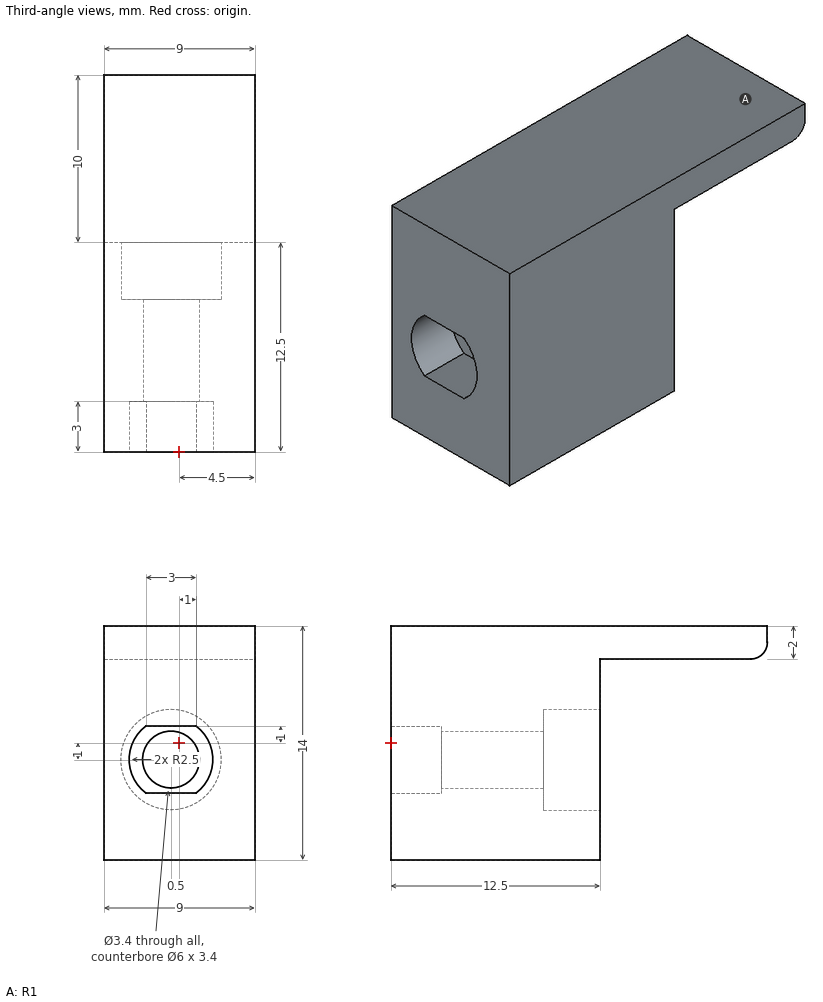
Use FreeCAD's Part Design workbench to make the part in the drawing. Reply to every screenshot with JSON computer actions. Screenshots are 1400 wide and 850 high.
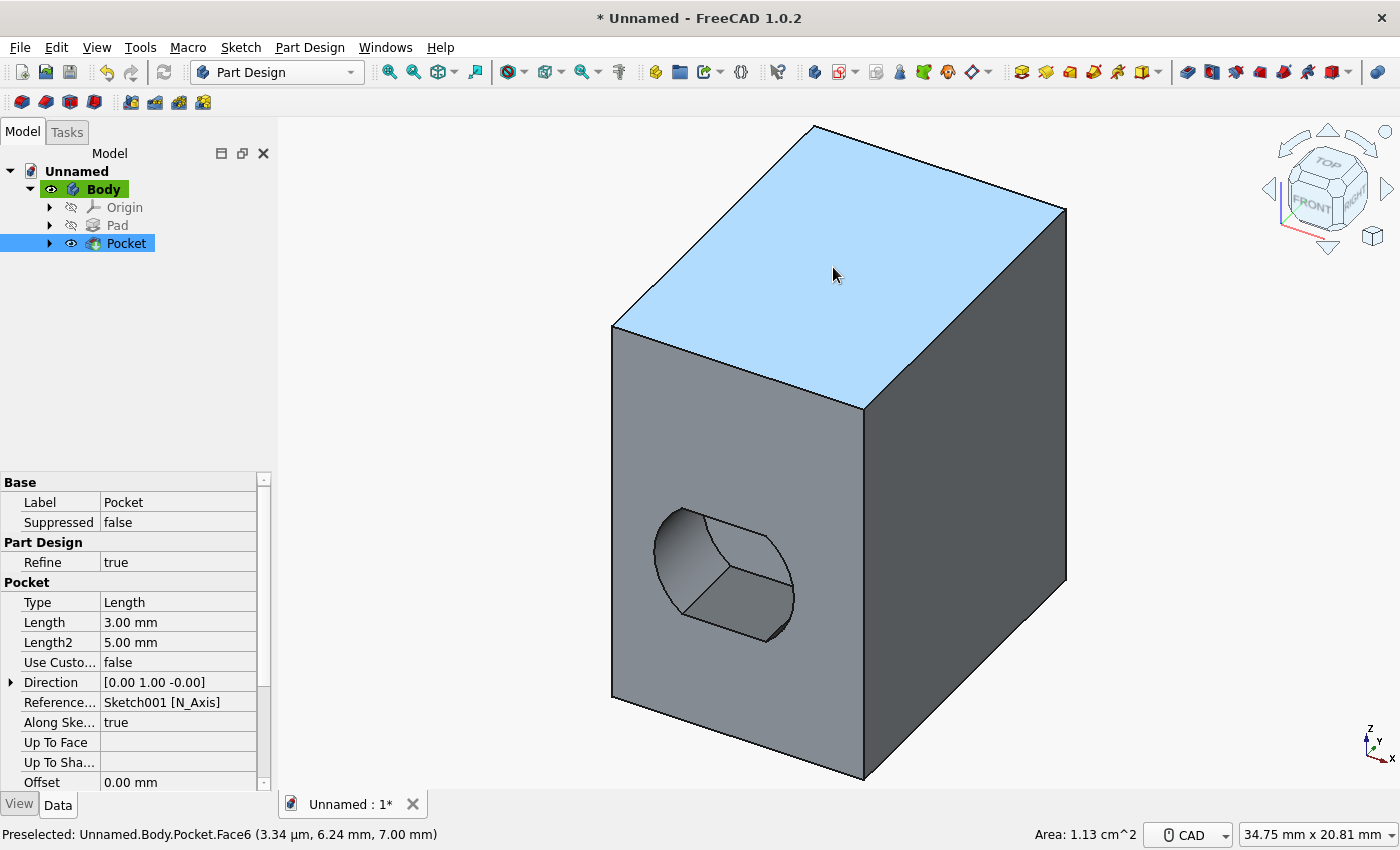
{"action": "left_click", "coordinate": [840, 72]}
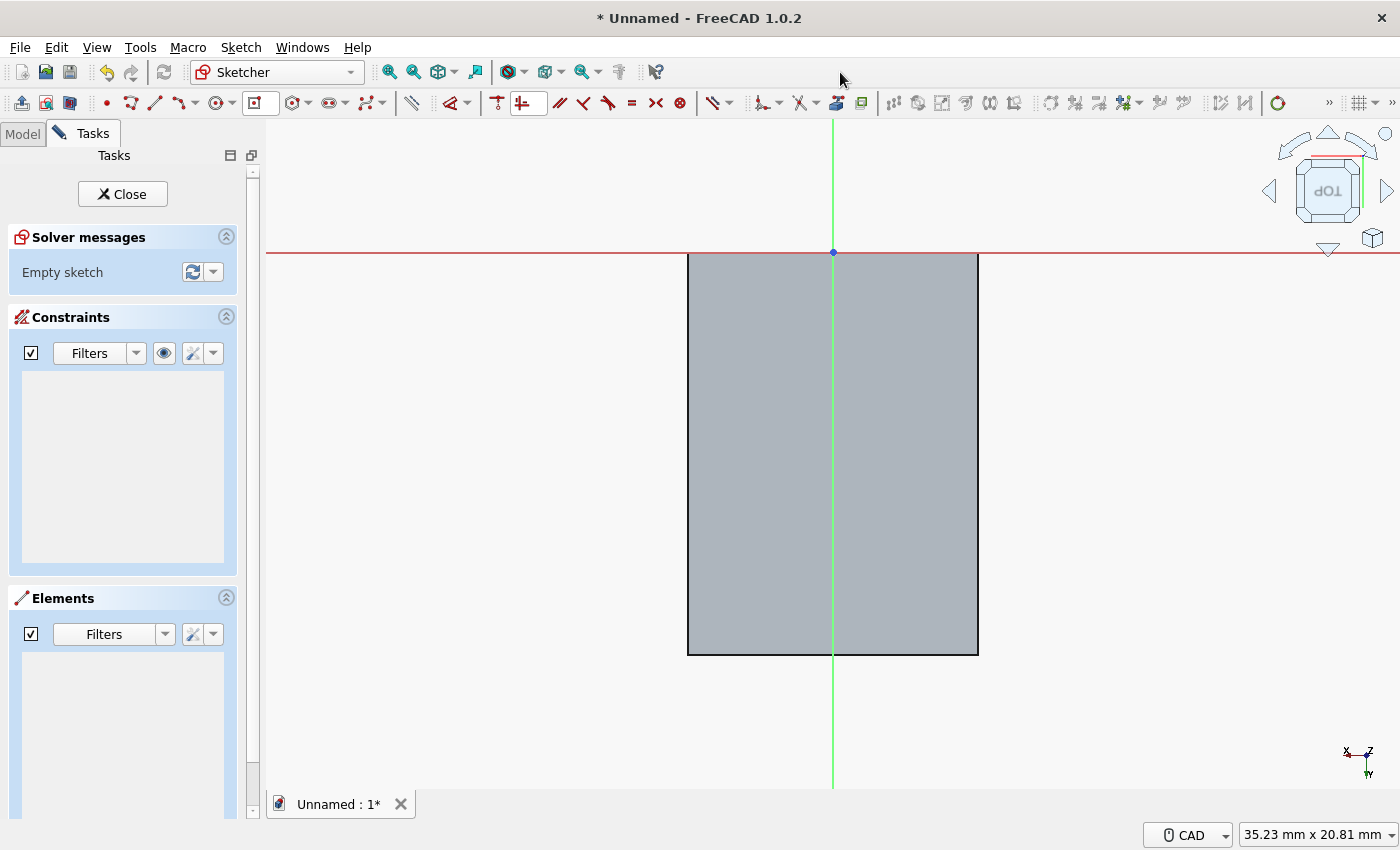
{"action": "scroll", "coordinate": [681, 258], "scroll_direction": "down", "scroll_amount": 3}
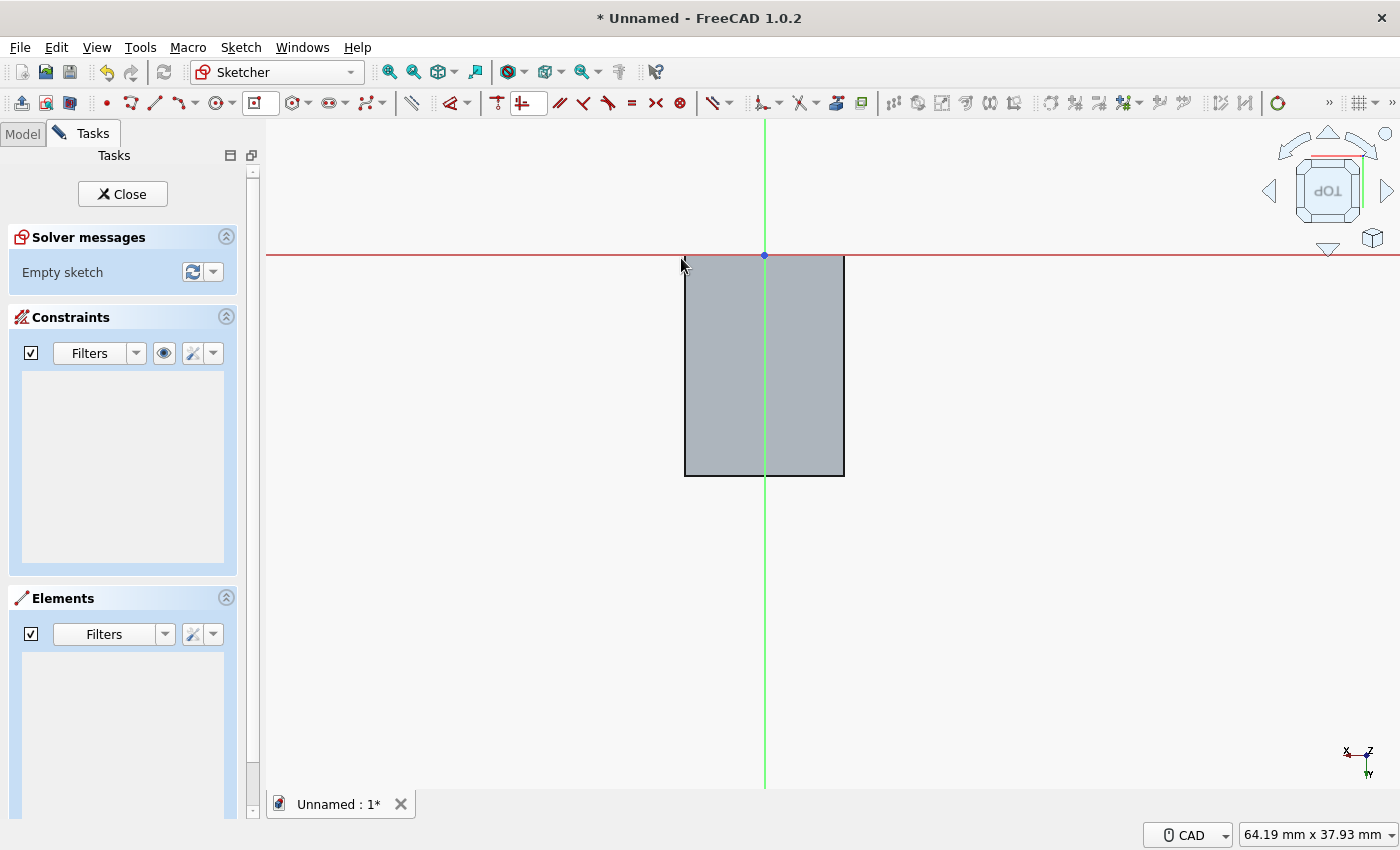
{"action": "key", "text": "g r"}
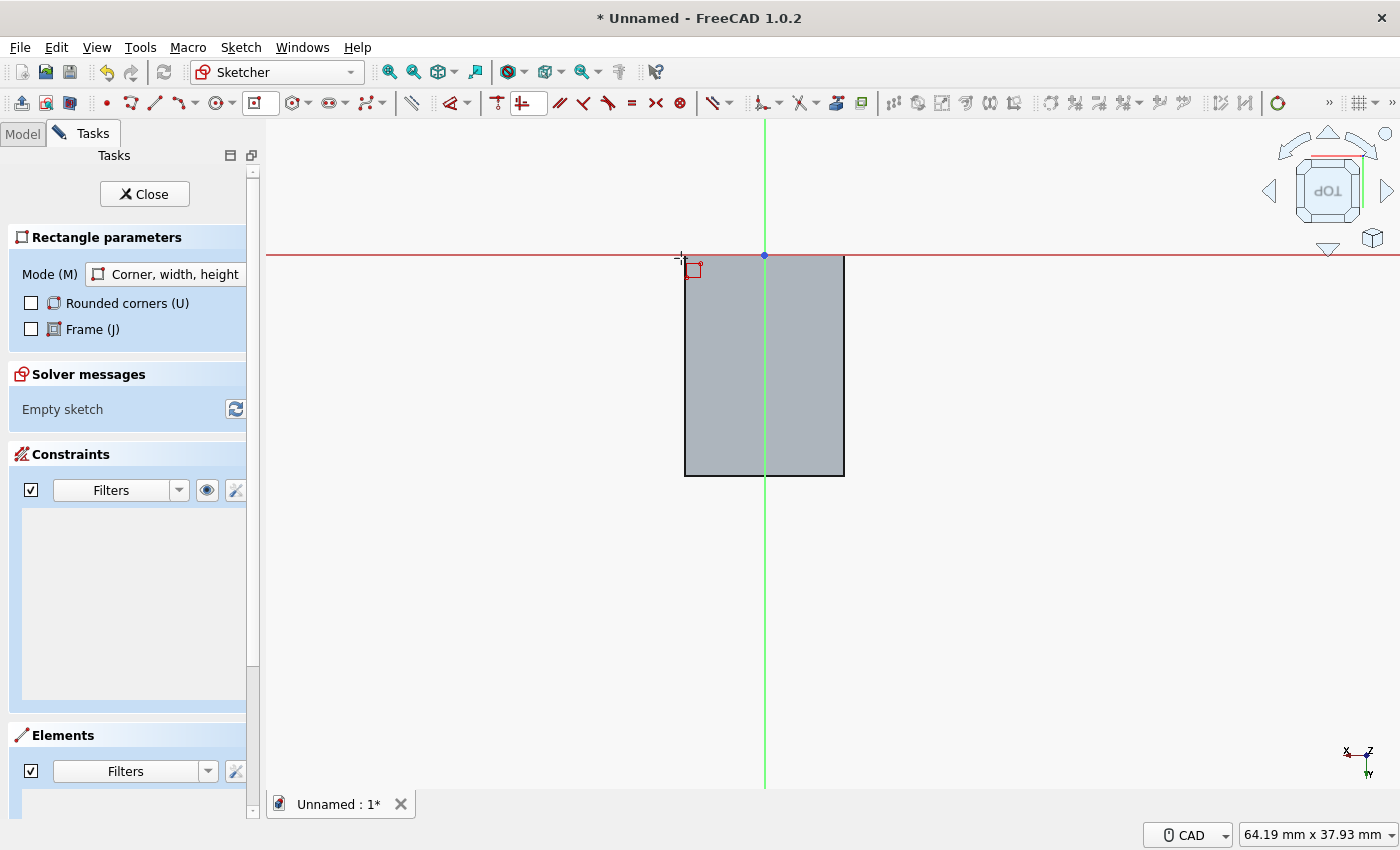
{"action": "left_click", "coordinate": [685, 476]}
{"action": "mouse_move", "coordinate": [844, 653]}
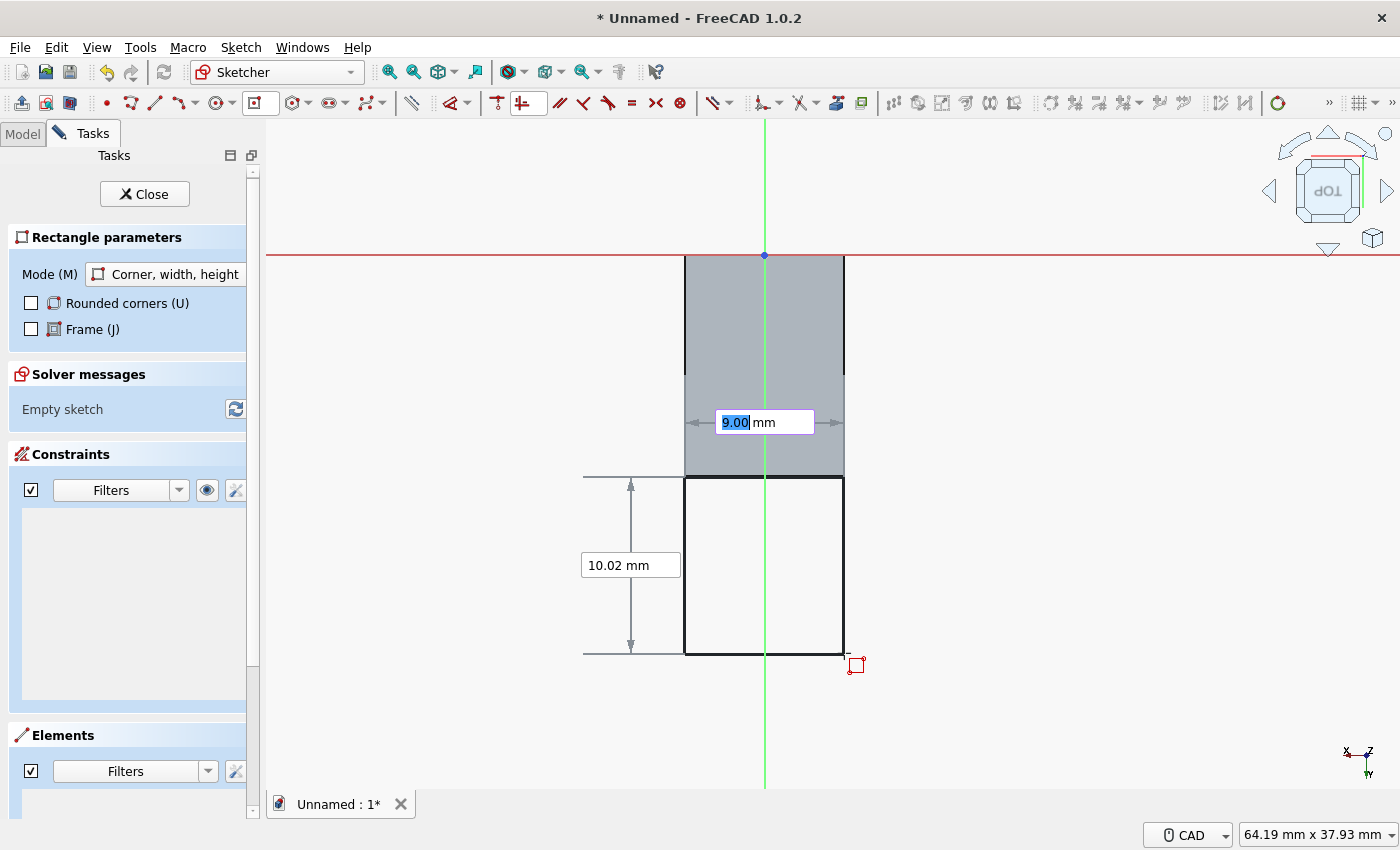
{"action": "type", "text": "9"}
{"action": "key", "text": "Tab"}
{"action": "type", "text": "10"}
{"action": "key", "text": "Return"}
{"action": "key", "text": "Escape"}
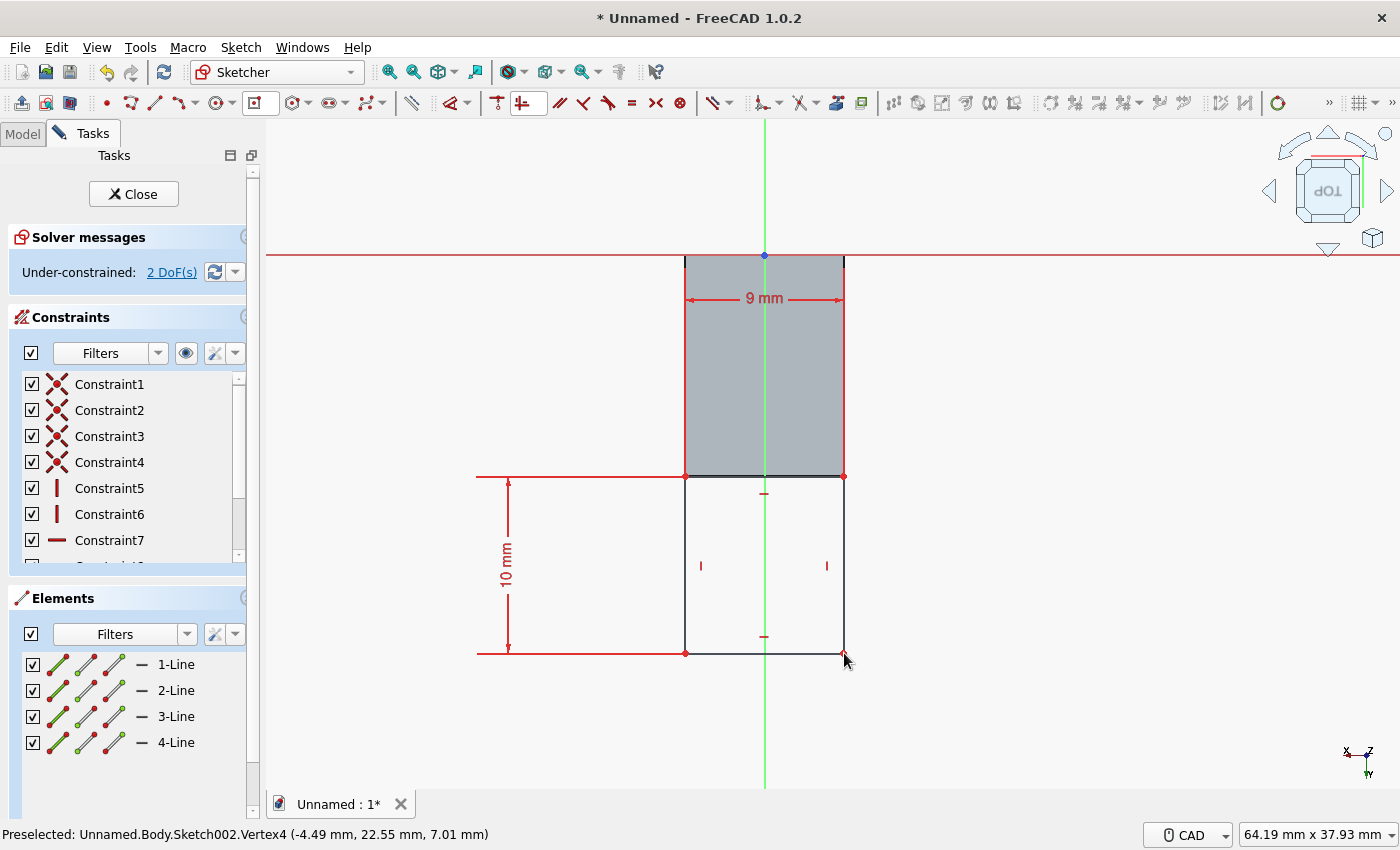
{"action": "left_click", "coordinate": [450, 104]}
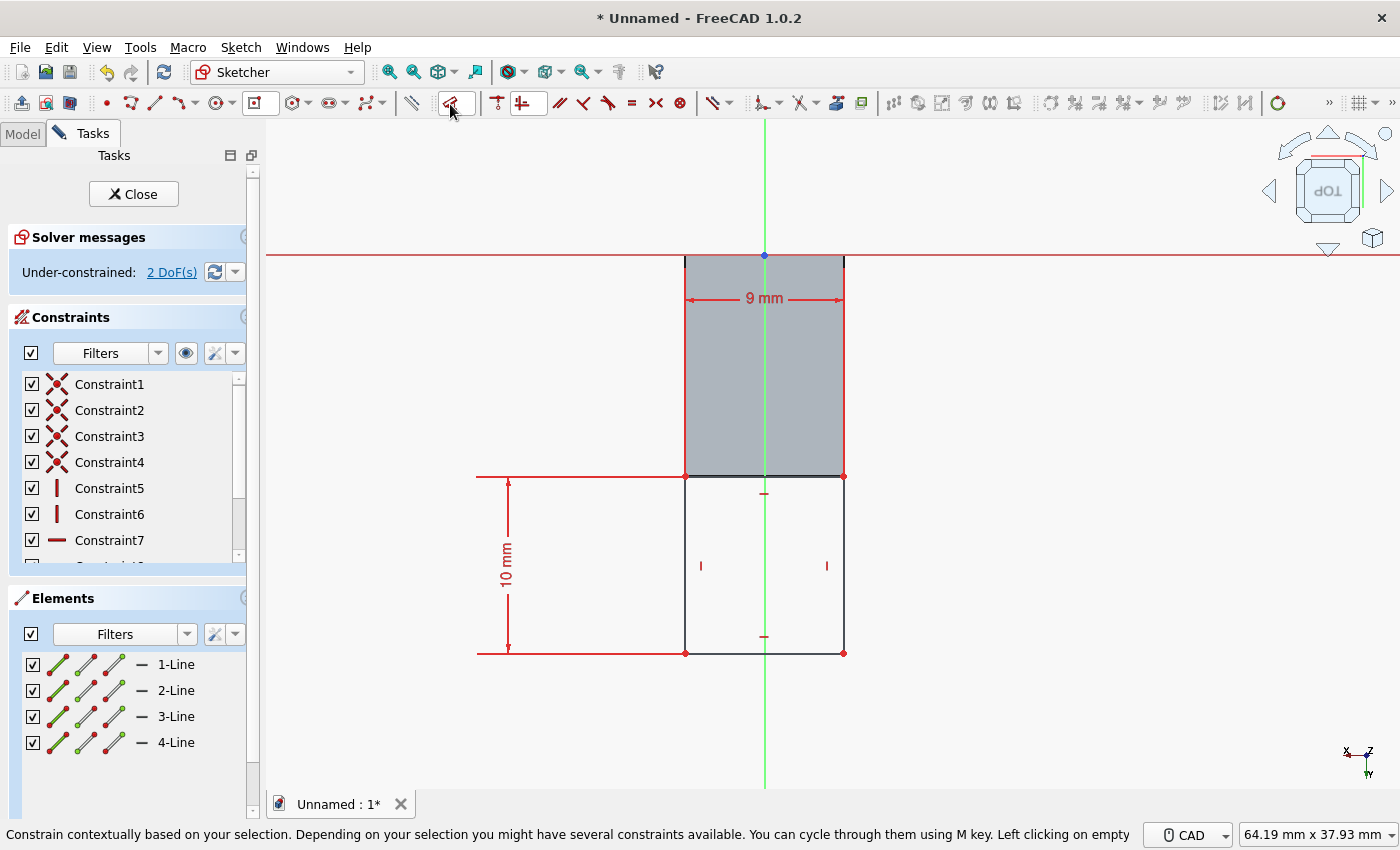
{"action": "left_click", "coordinate": [685, 477]}
{"action": "left_click", "coordinate": [725, 221]}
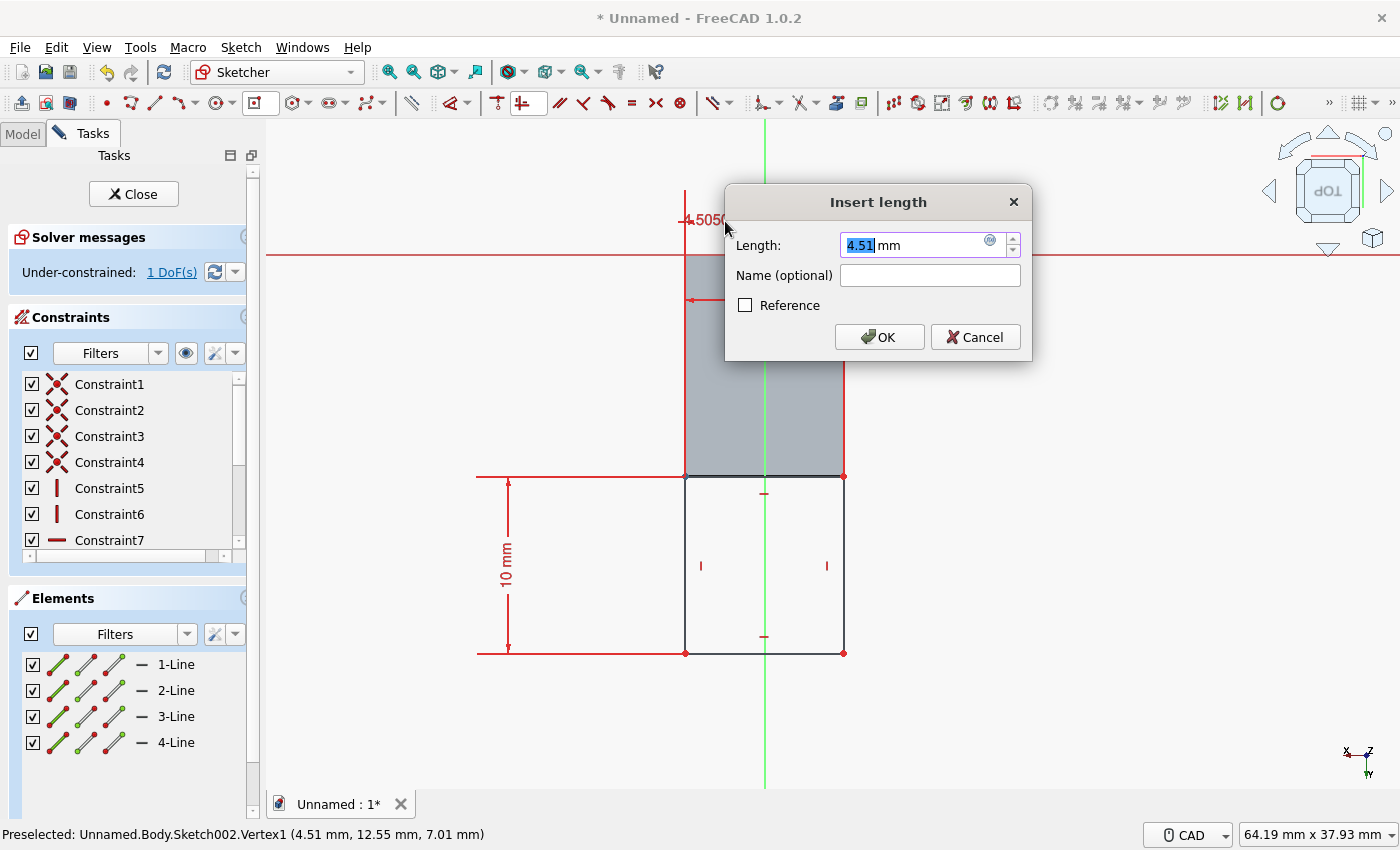
{"action": "type", "text": "4.5"}
{"action": "key", "text": "Return"}